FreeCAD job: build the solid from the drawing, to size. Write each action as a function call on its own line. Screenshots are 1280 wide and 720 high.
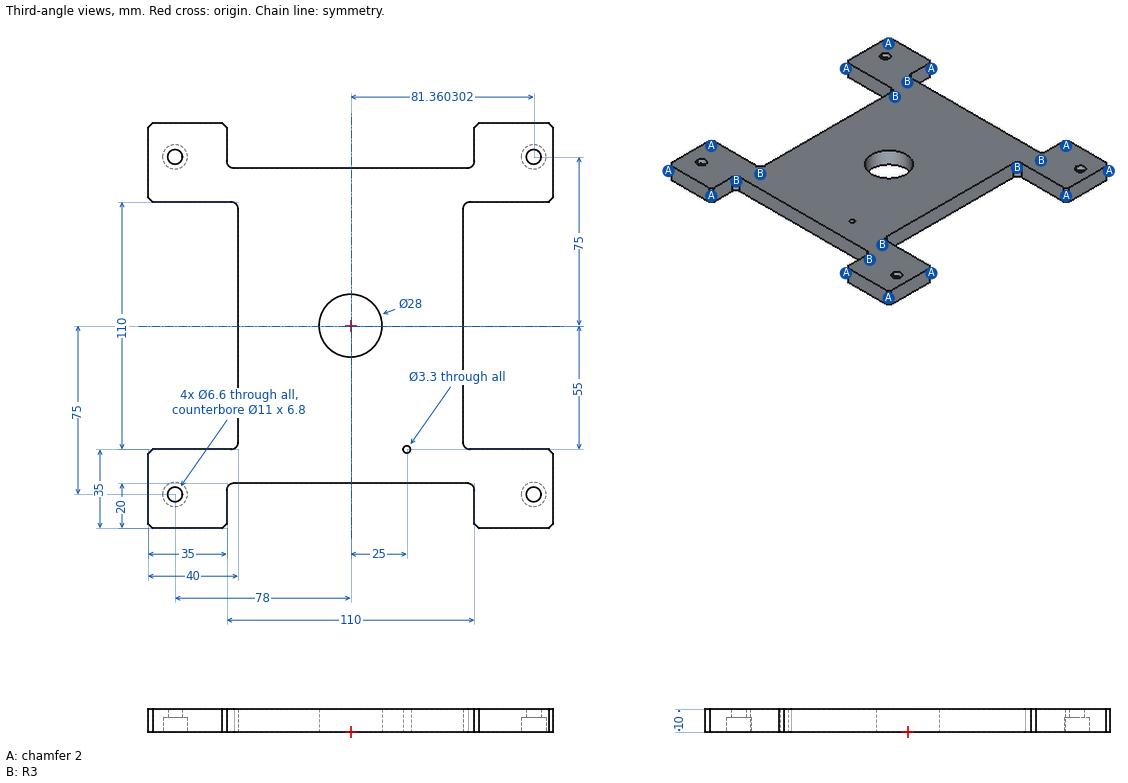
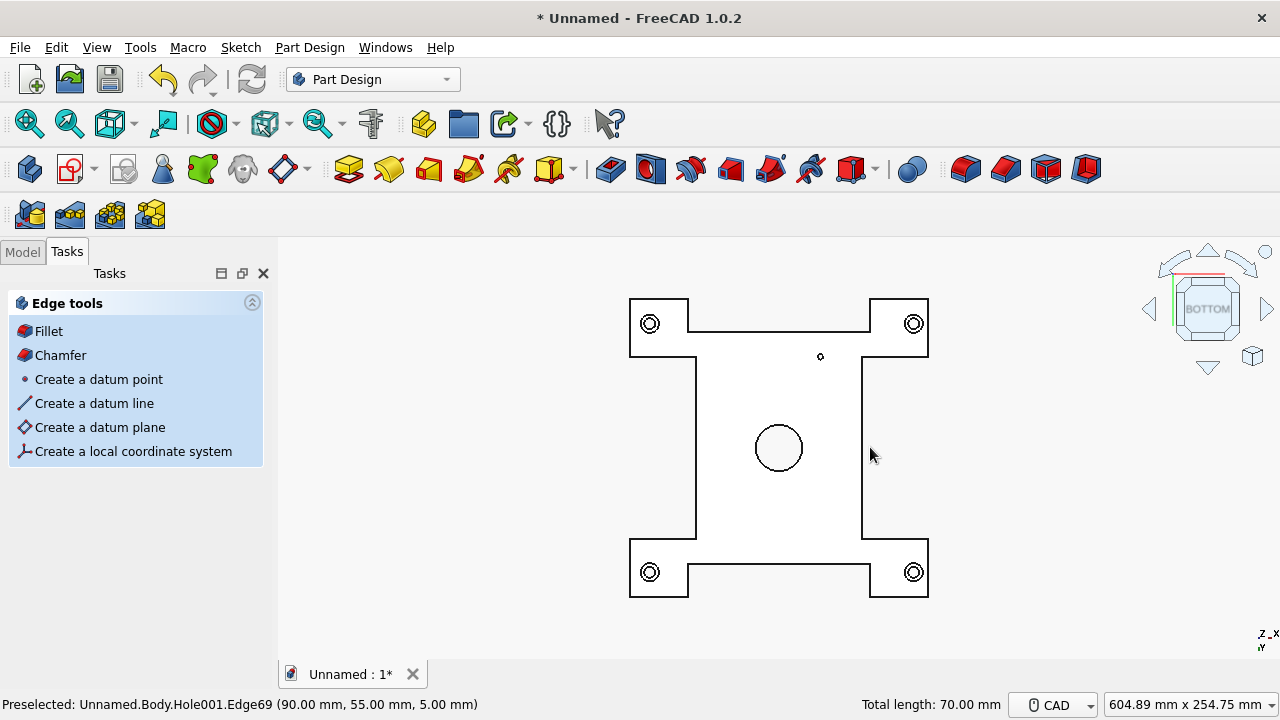
scroll(630, 538, up, 5)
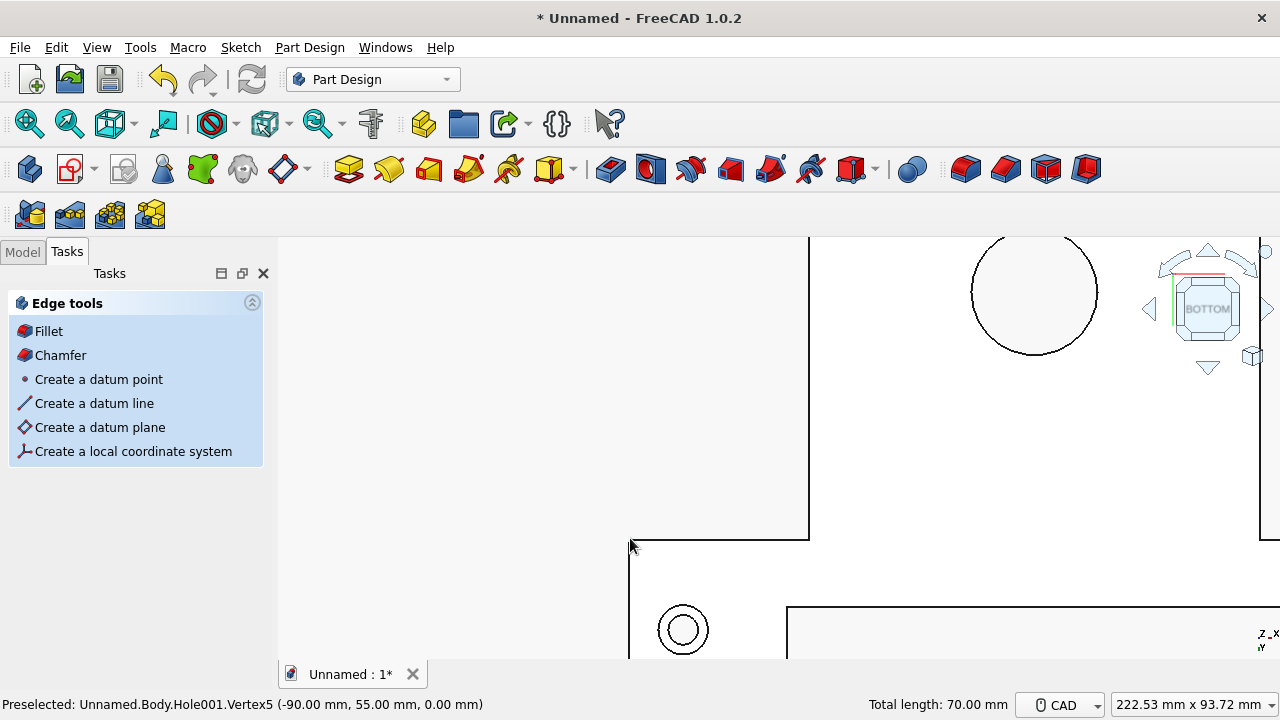
click(30, 124)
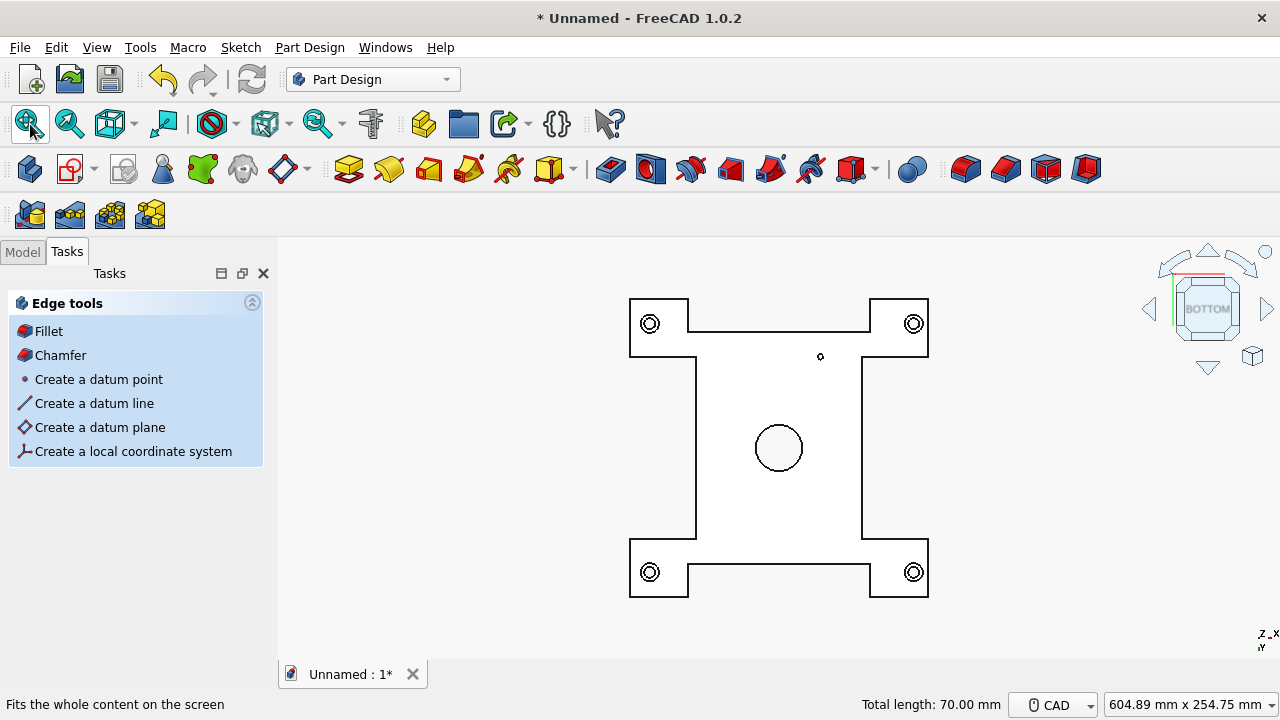
key(4)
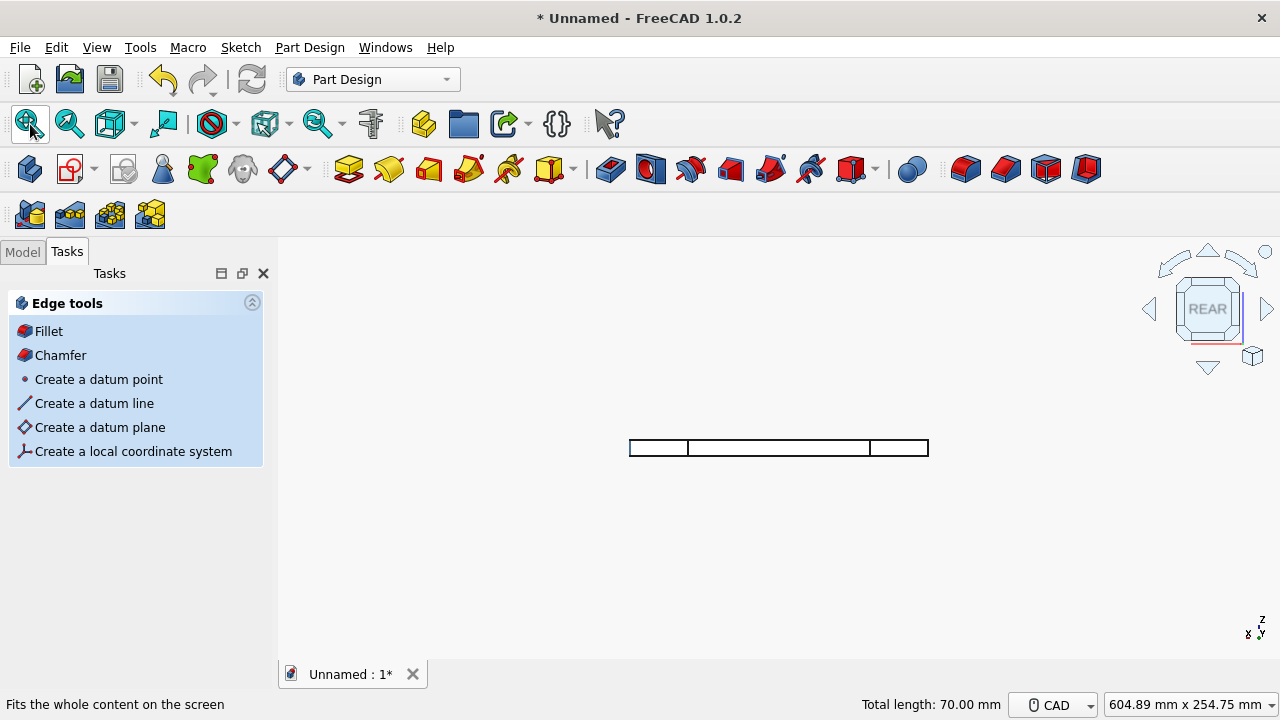
click(30, 124)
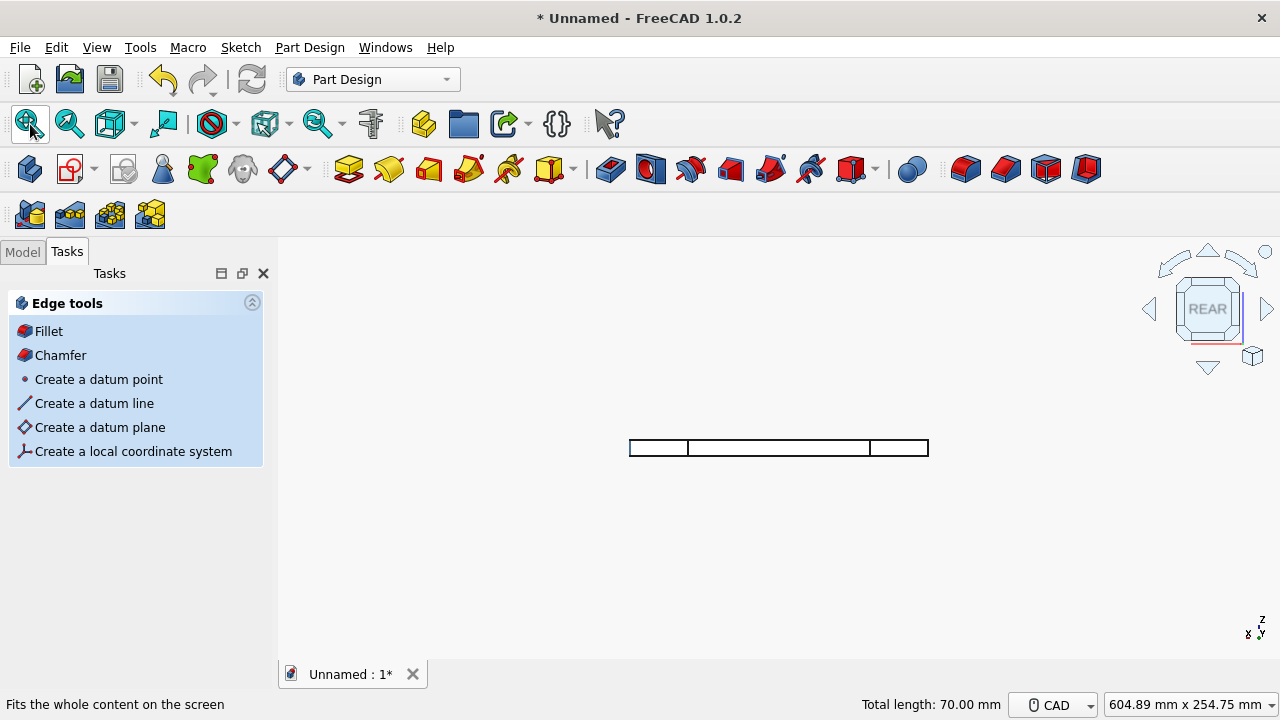
click(928, 447, ctrl)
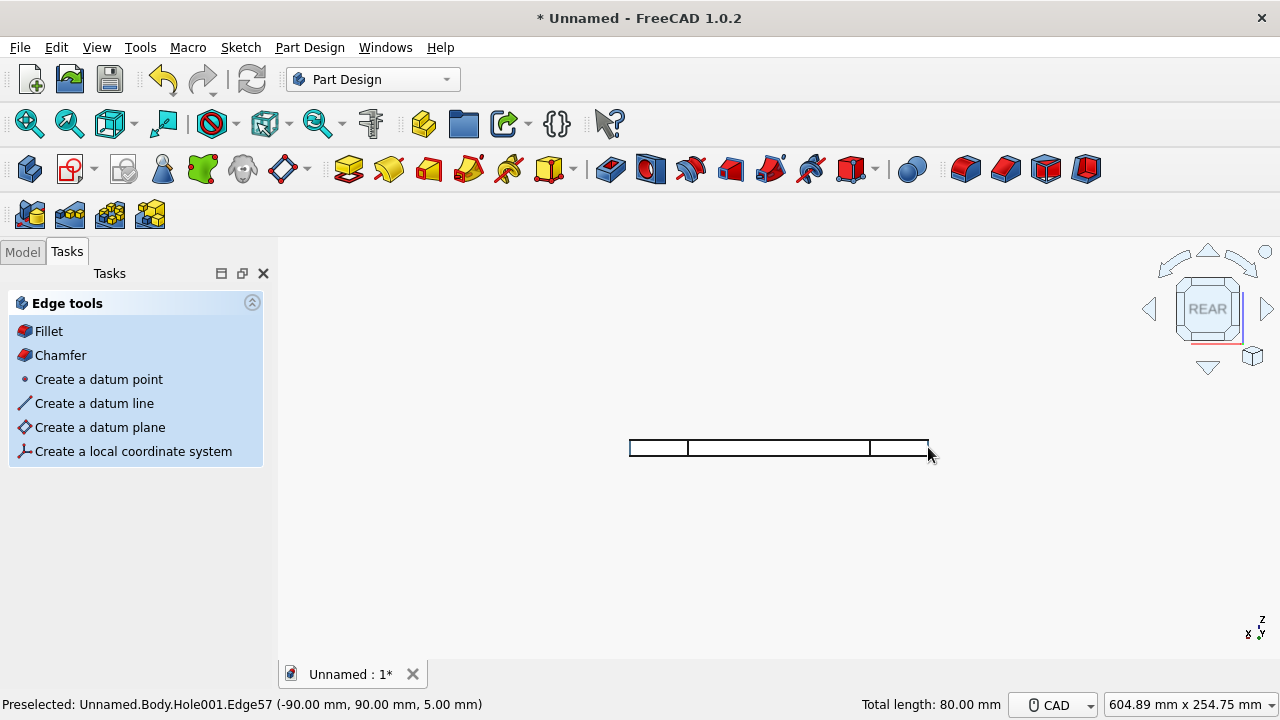
click(870, 447, ctrl)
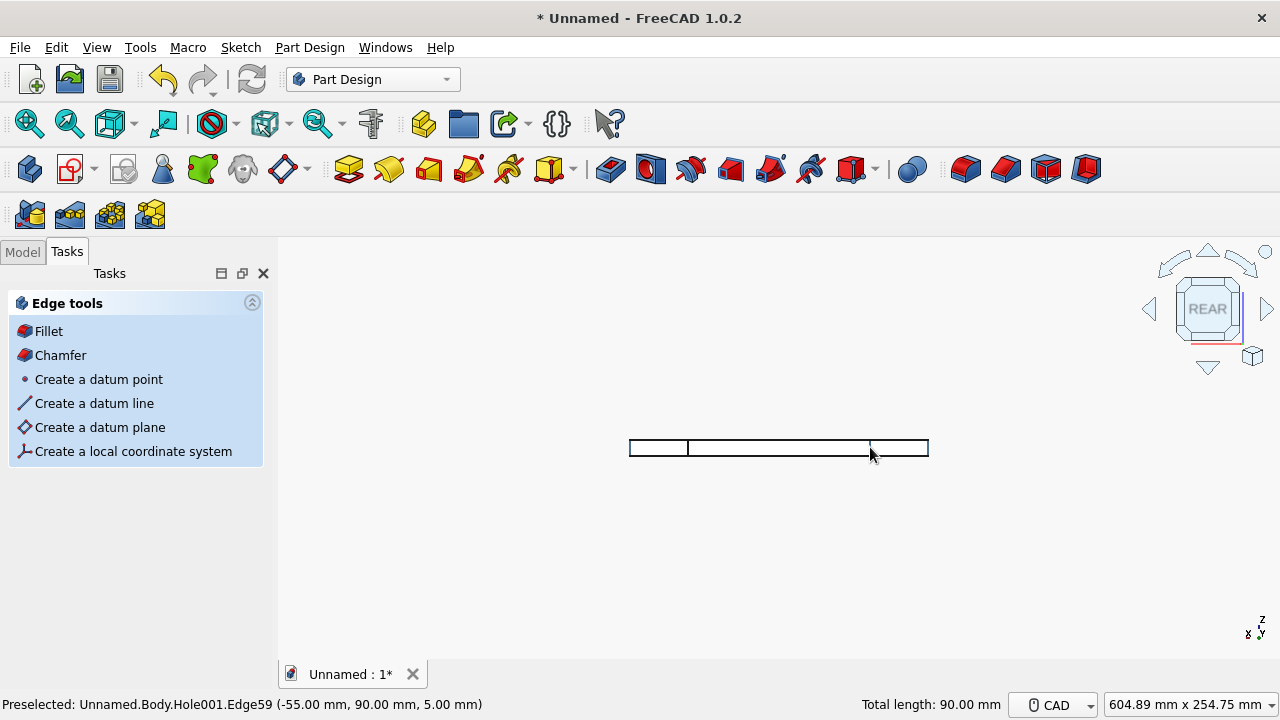
click(688, 447, ctrl)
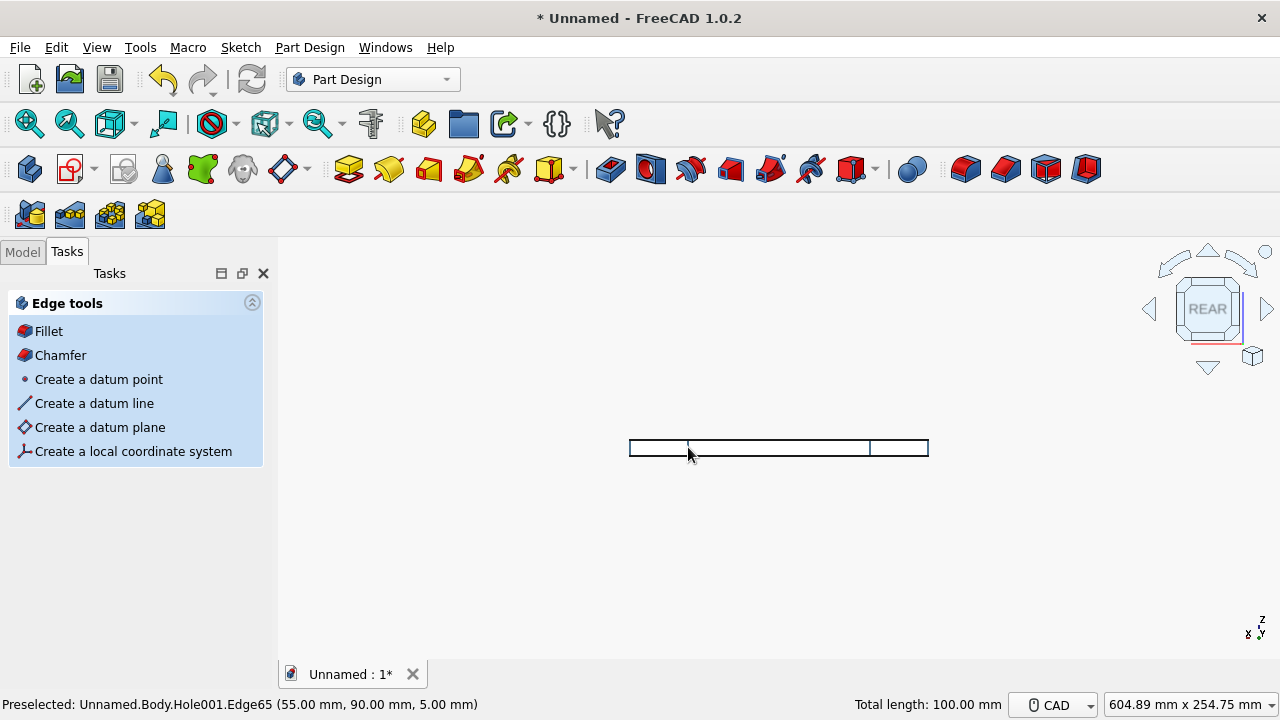
scroll(928, 447, up, 5)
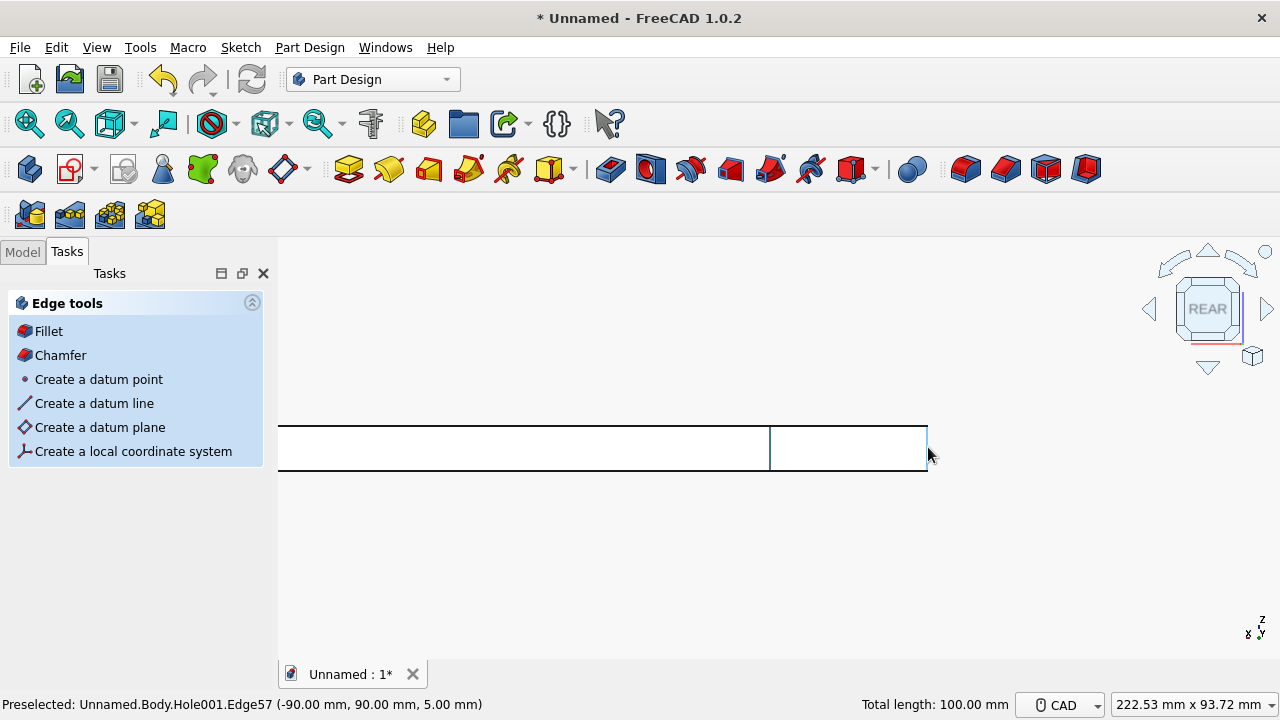
click(30, 124)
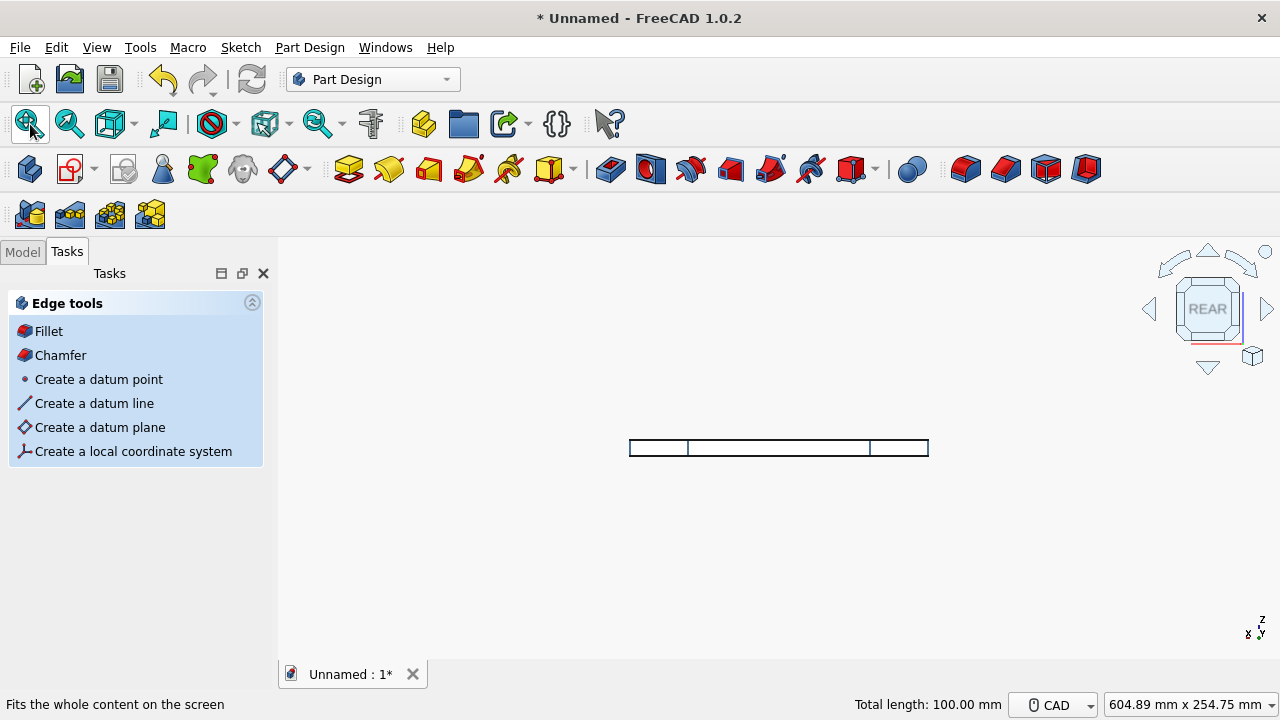
key(6)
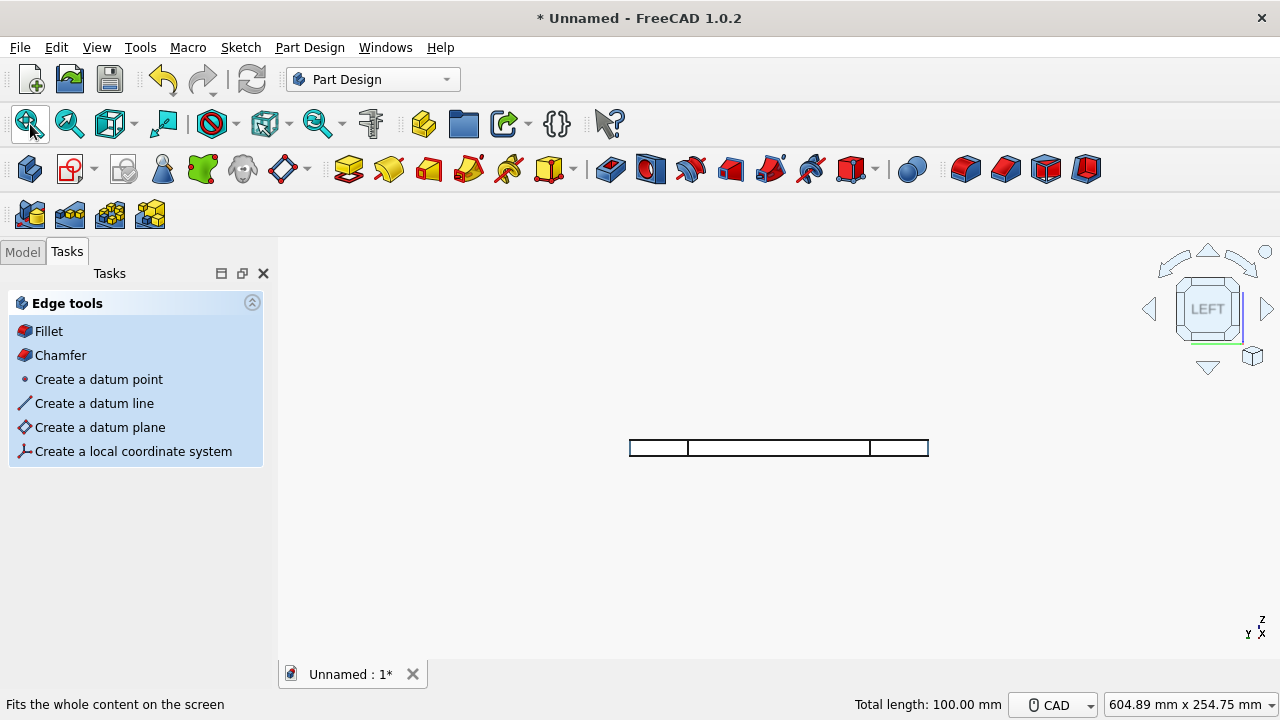
click(30, 124)